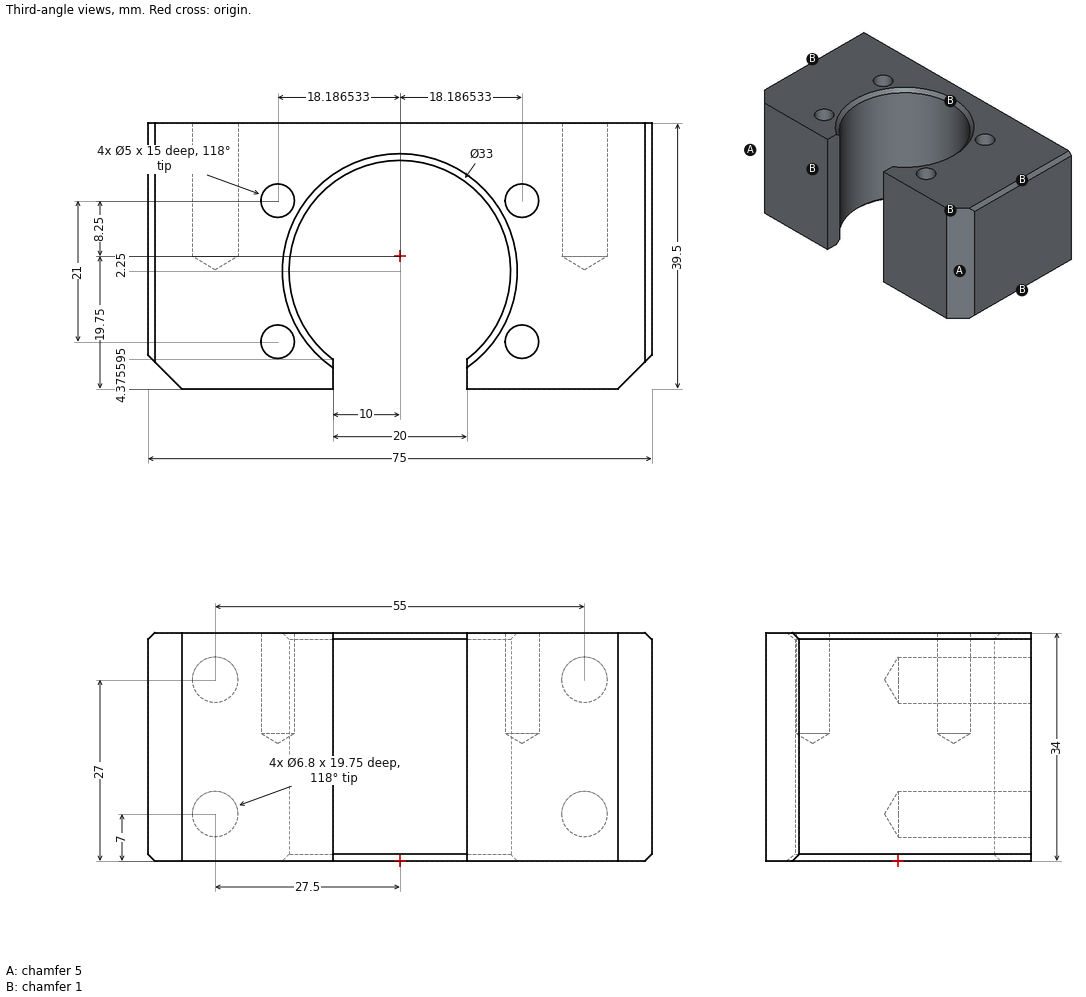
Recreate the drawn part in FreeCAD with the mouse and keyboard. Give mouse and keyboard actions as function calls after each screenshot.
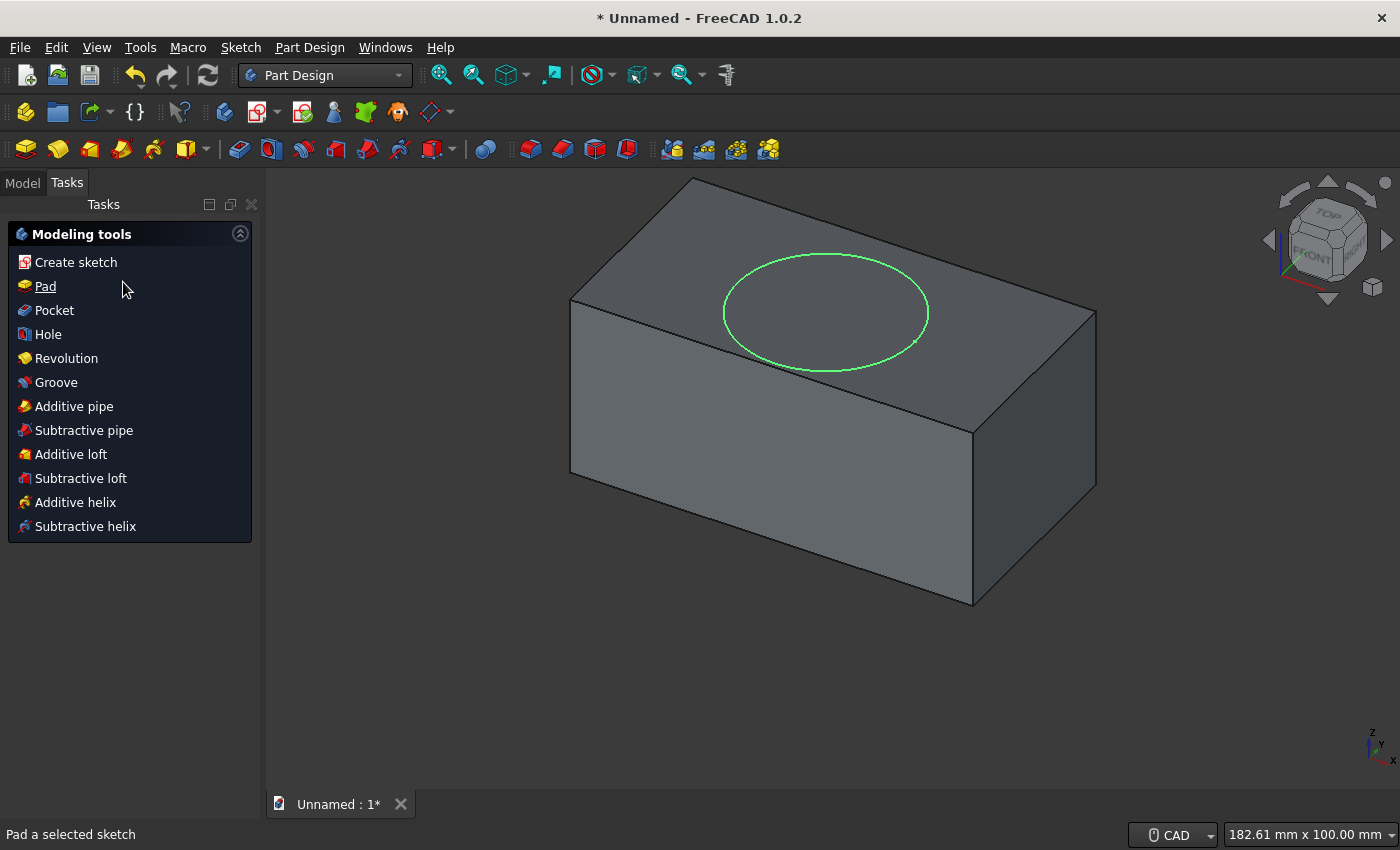
click(240, 150)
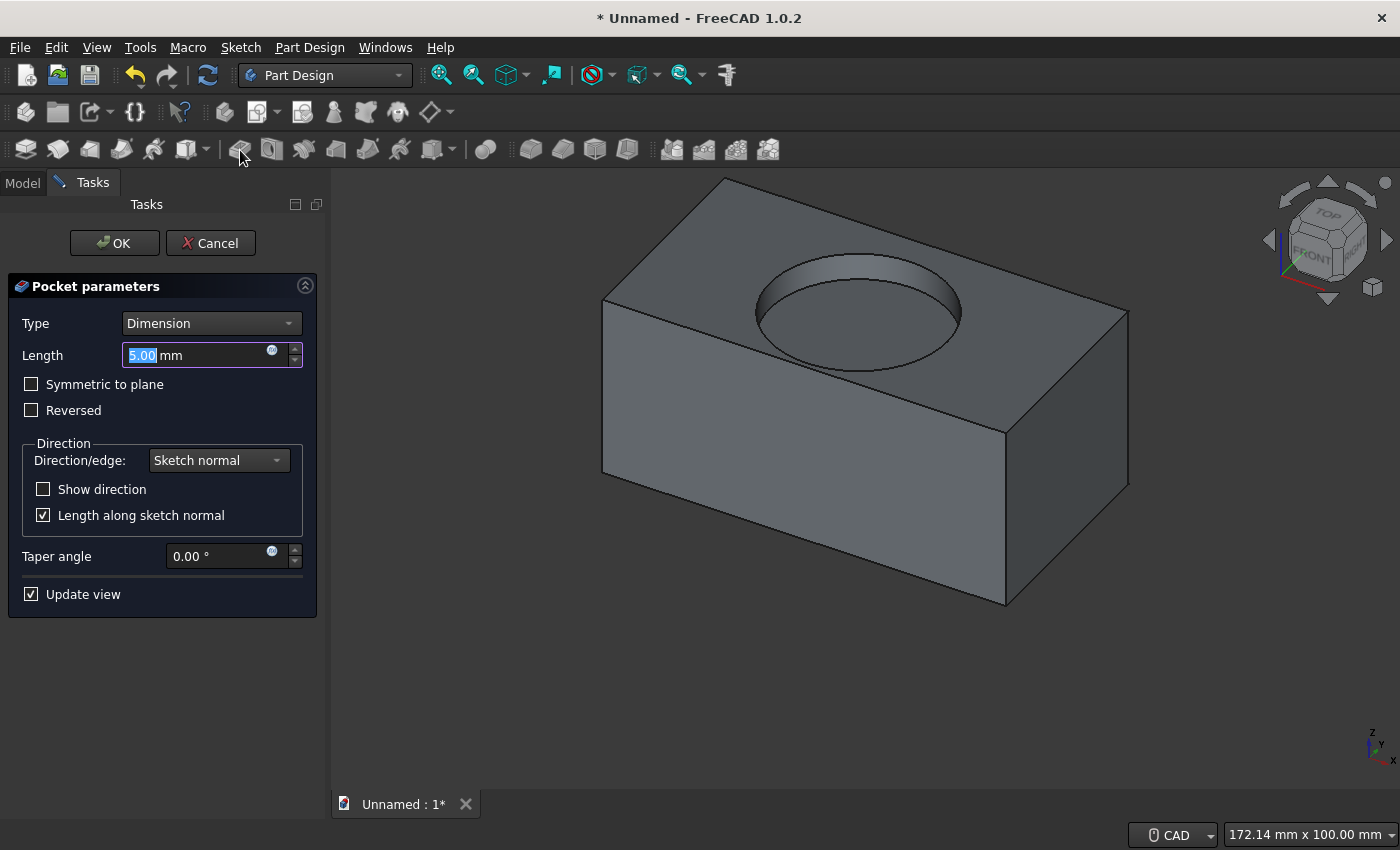
click(212, 324)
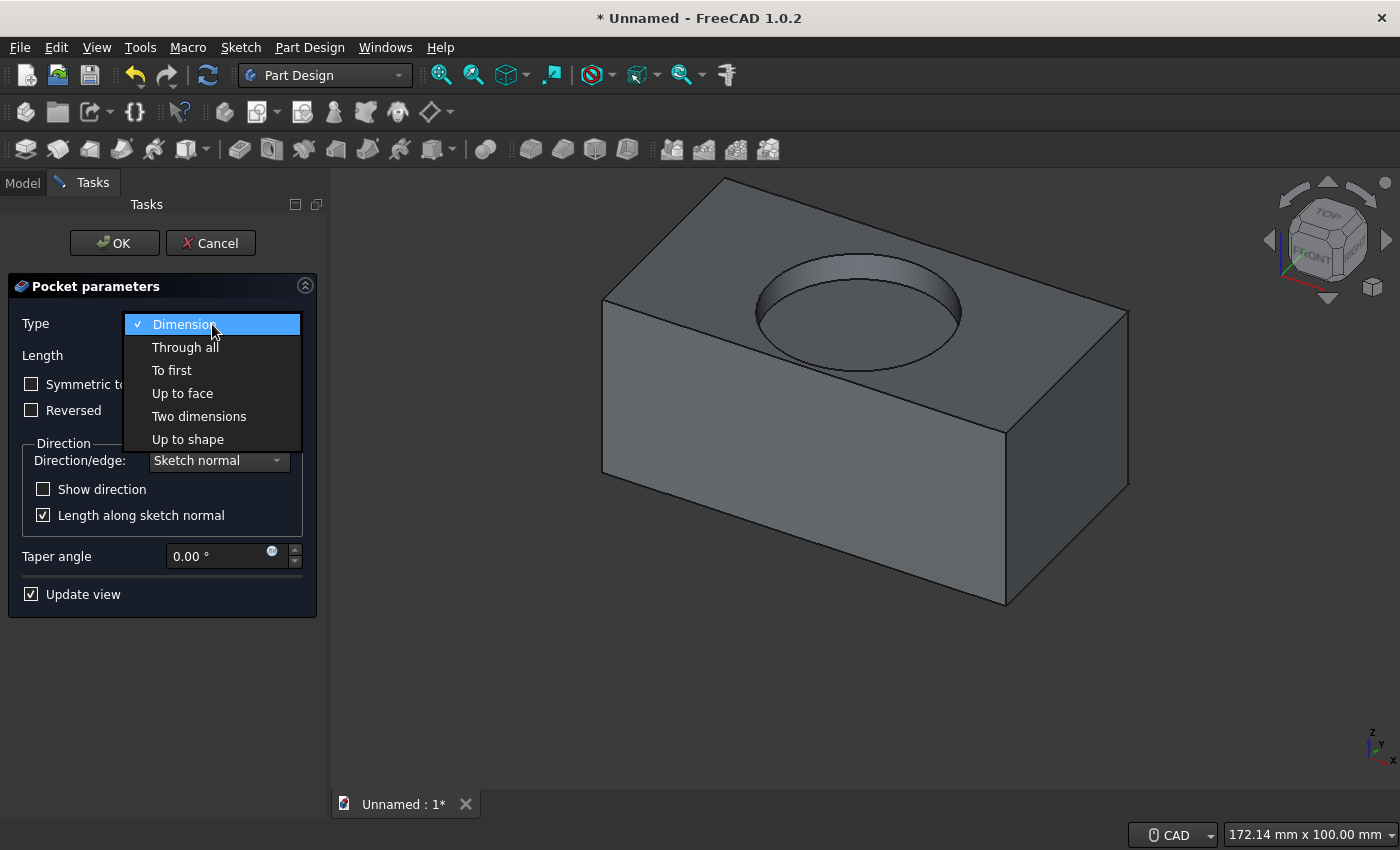
click(212, 348)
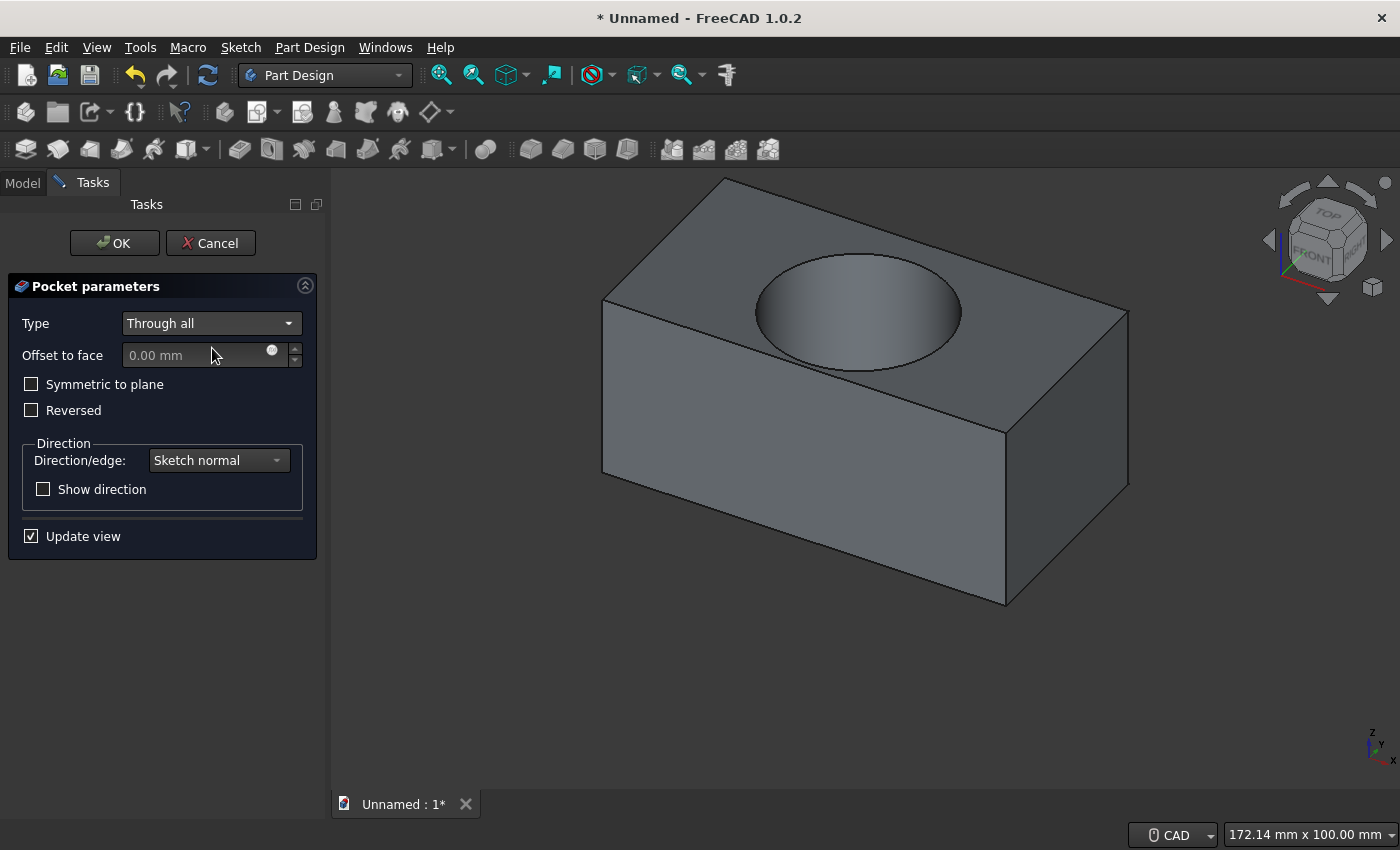
click(115, 243)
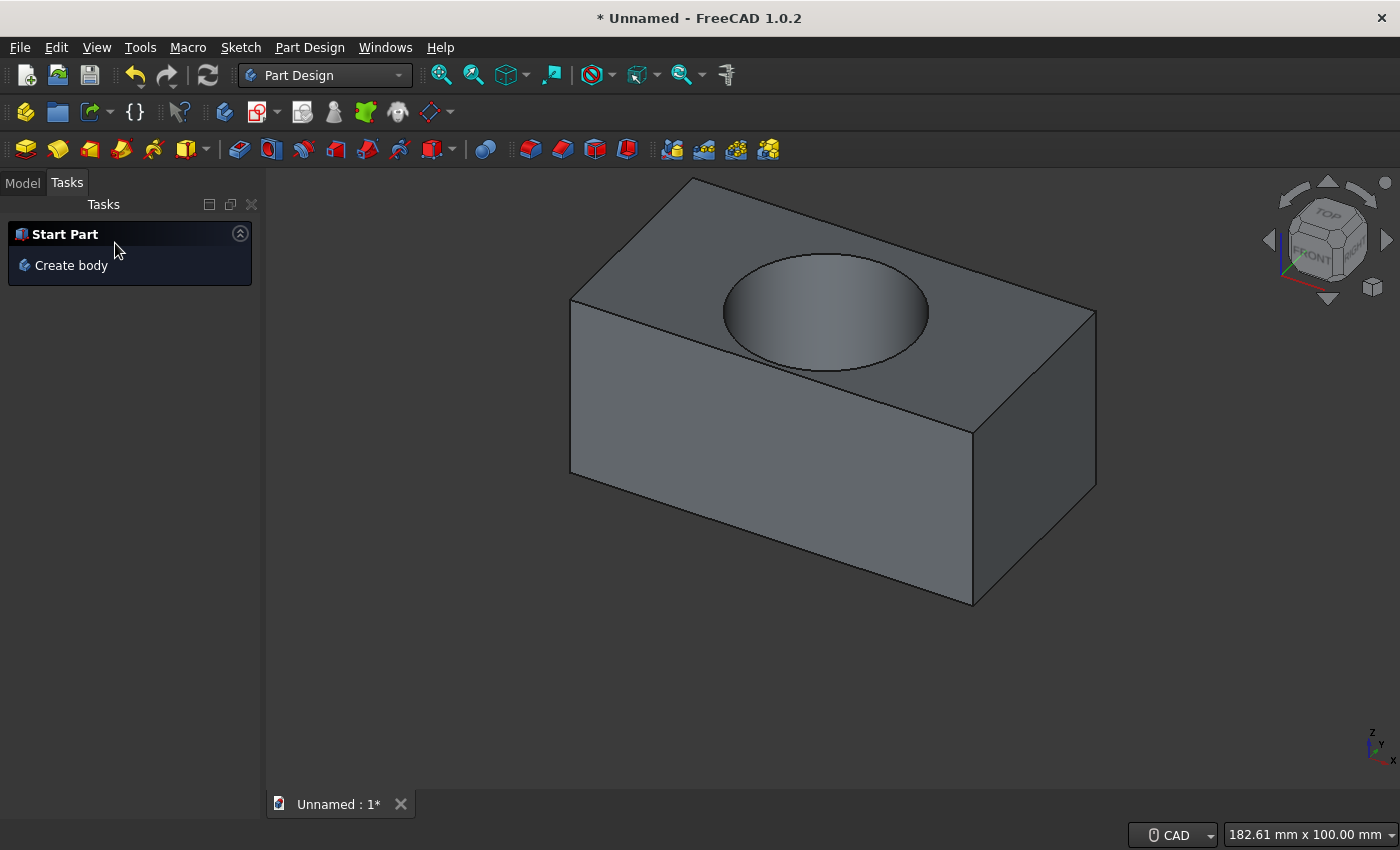
click(983, 308)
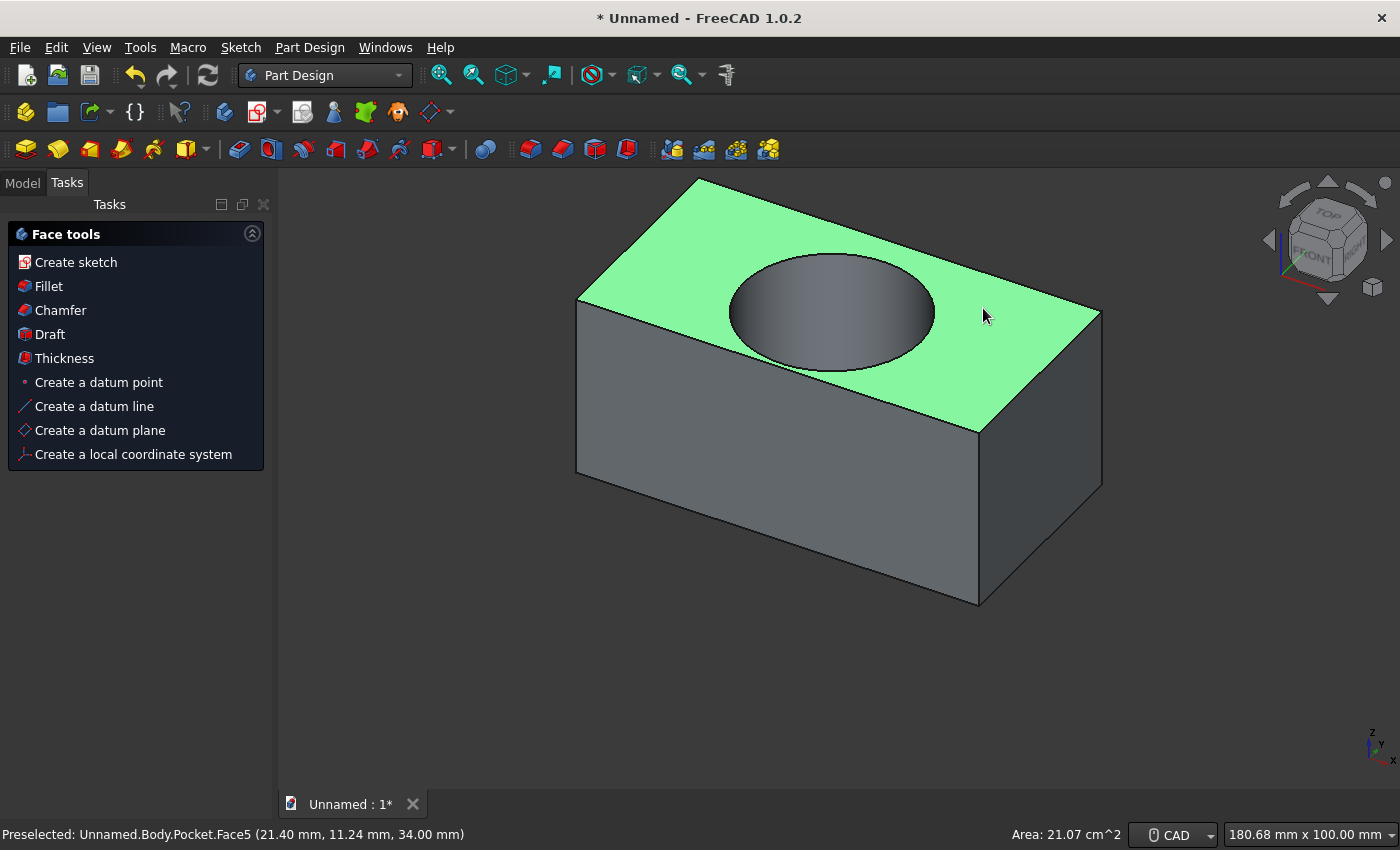
click(258, 112)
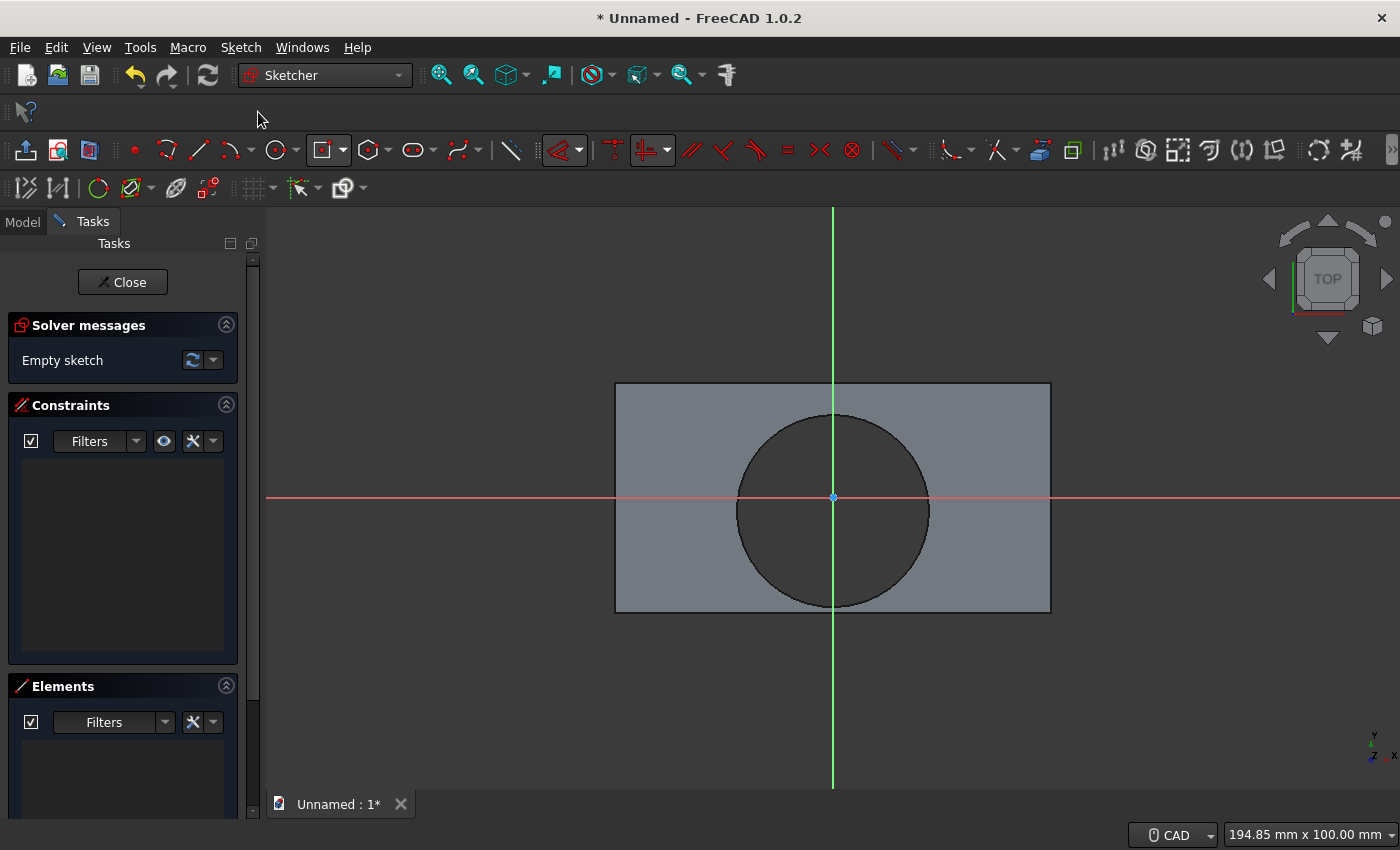
scroll(863, 580, up, 6)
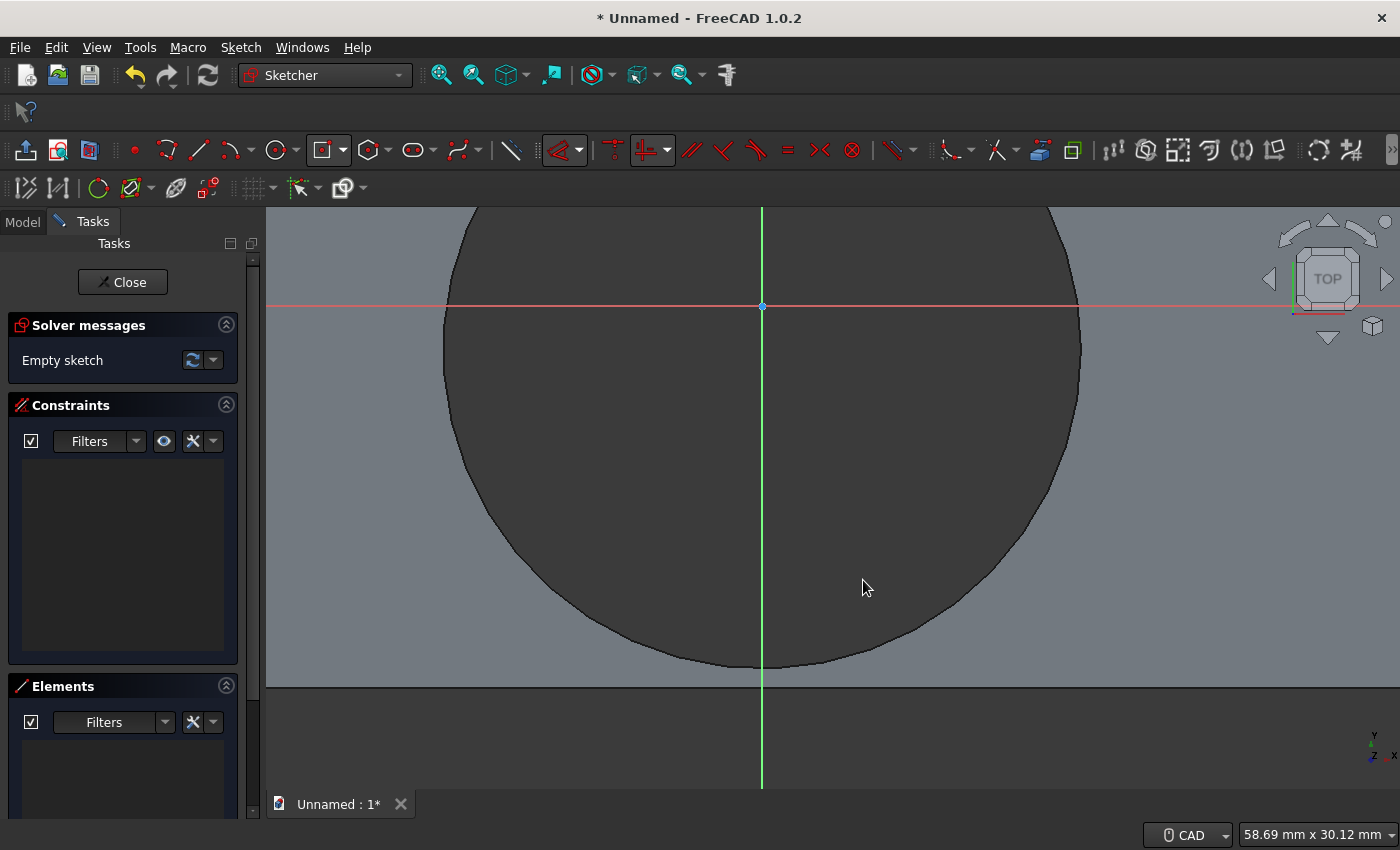
click(346, 150)